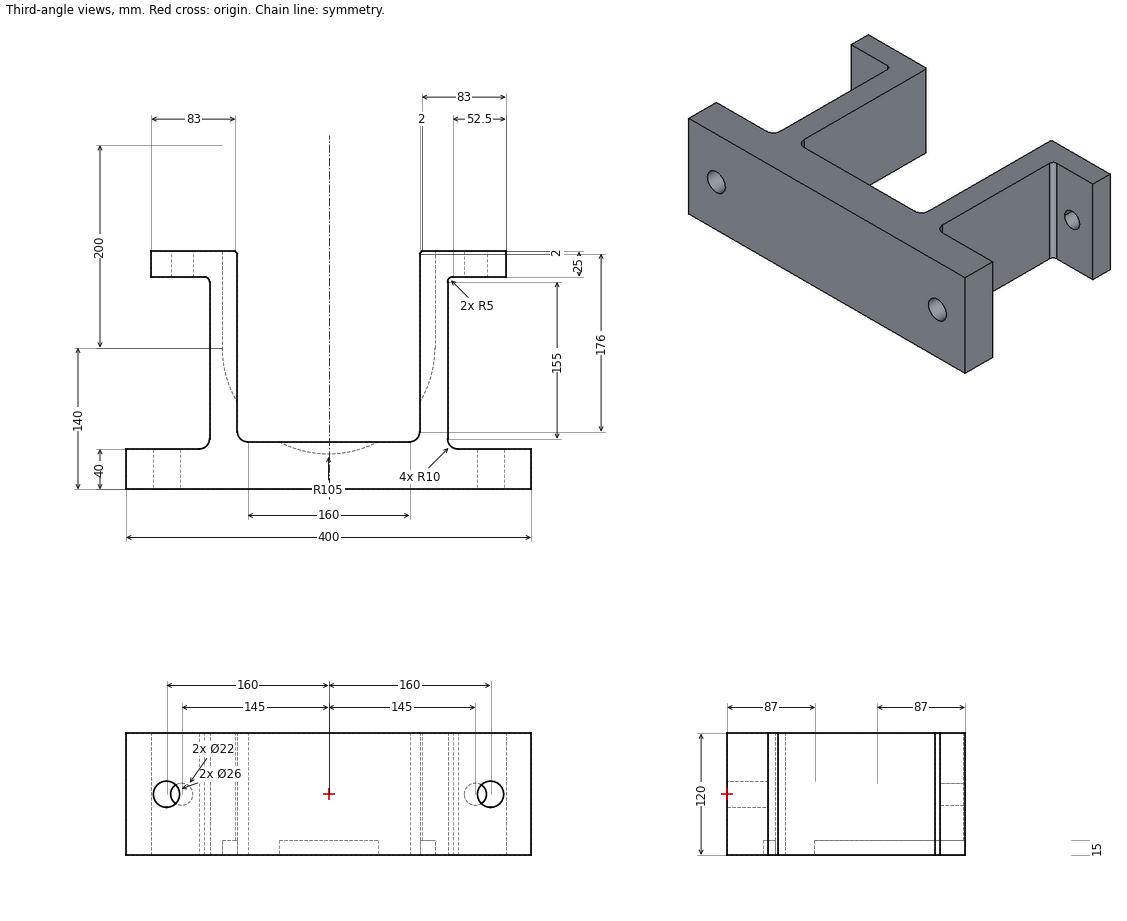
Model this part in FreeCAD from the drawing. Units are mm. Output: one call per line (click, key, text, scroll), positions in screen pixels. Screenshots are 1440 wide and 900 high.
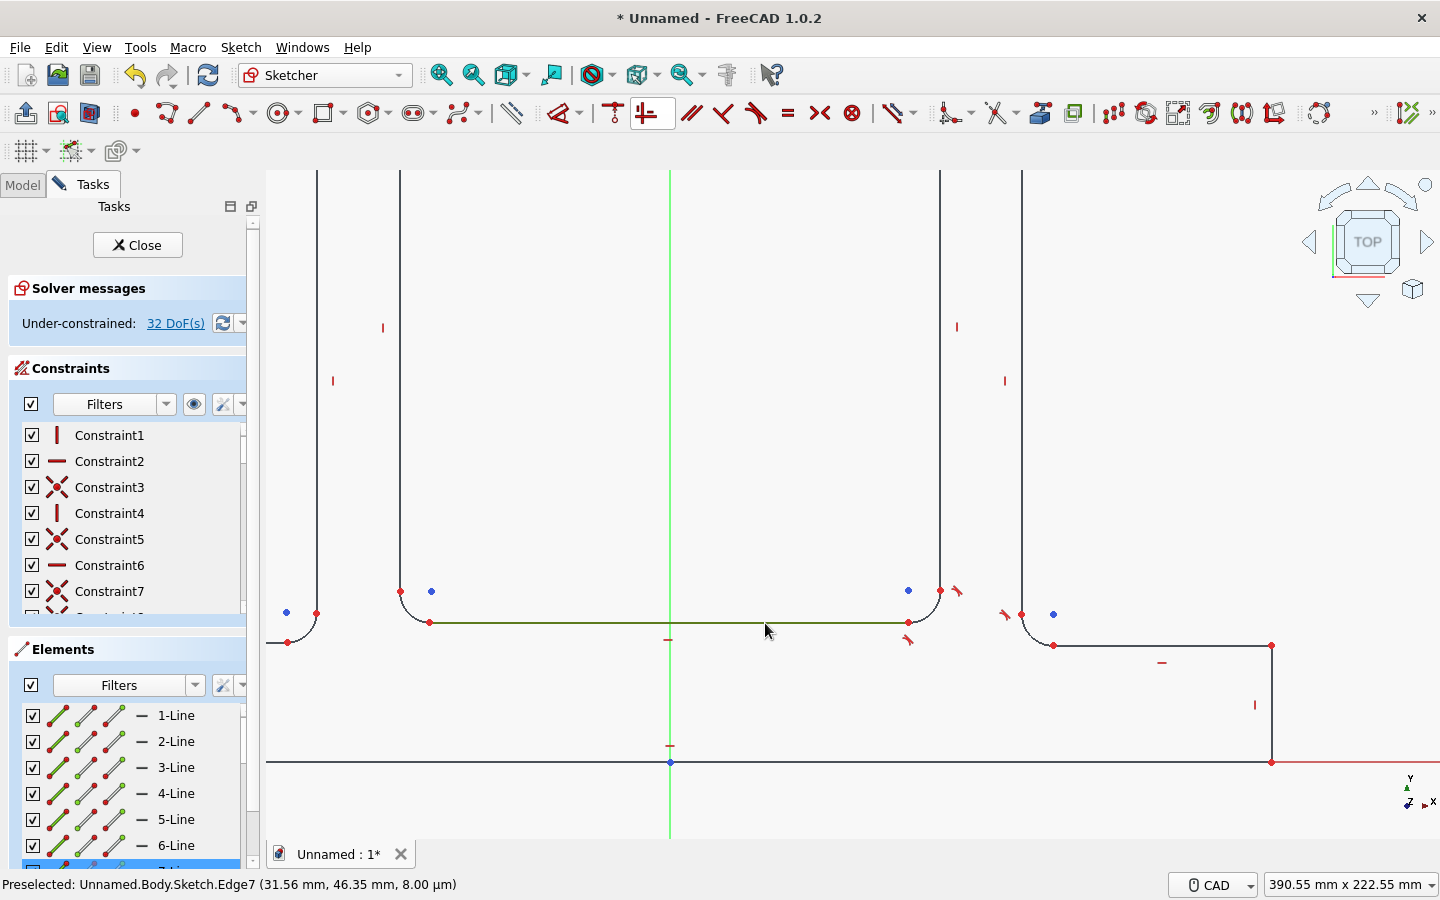
click(403, 605)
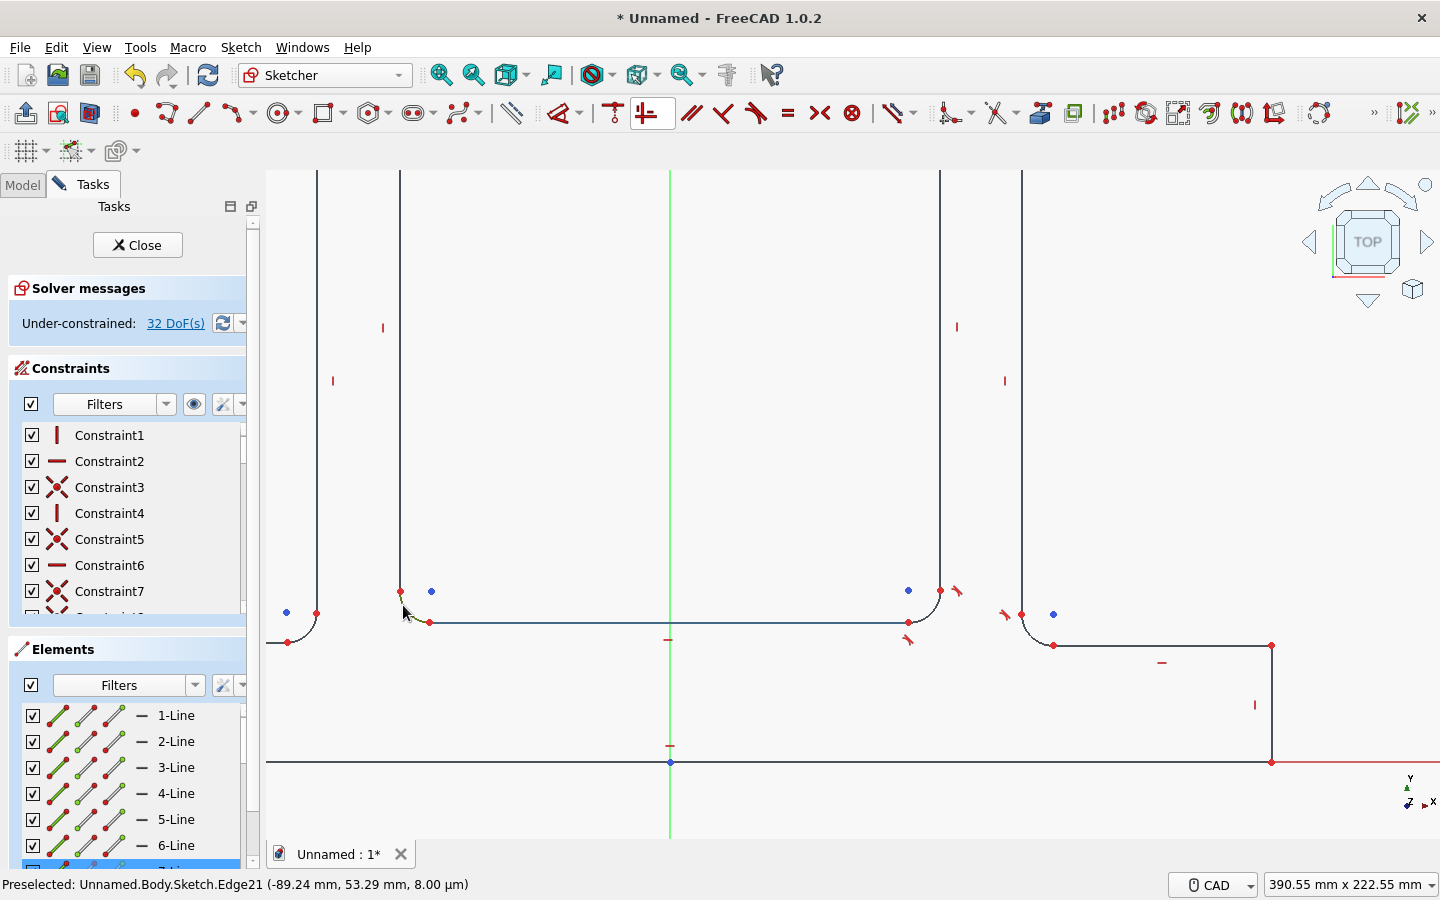
click(756, 114)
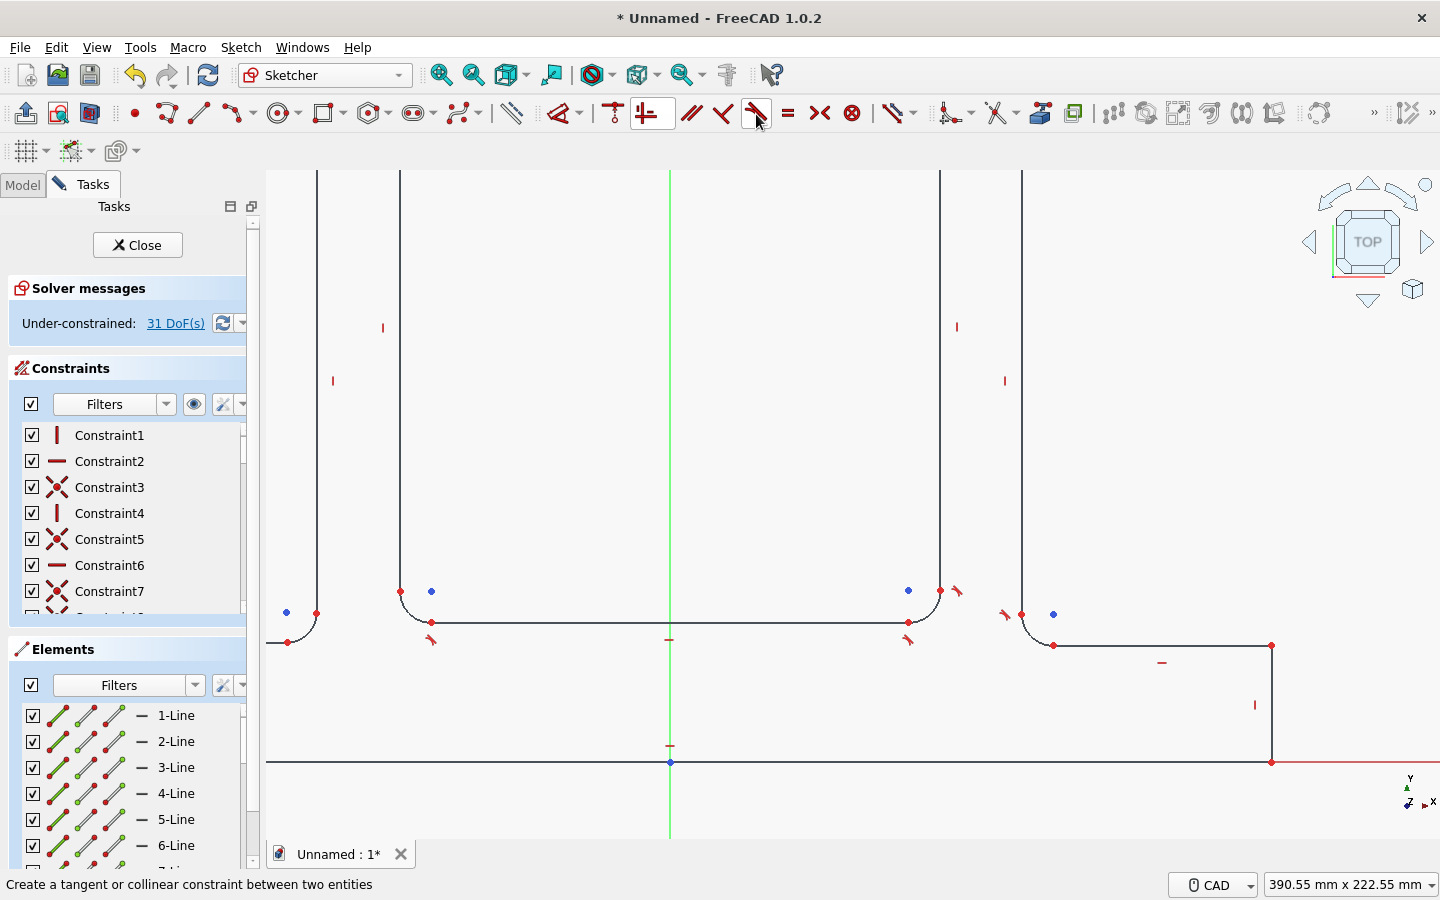
click(400, 433)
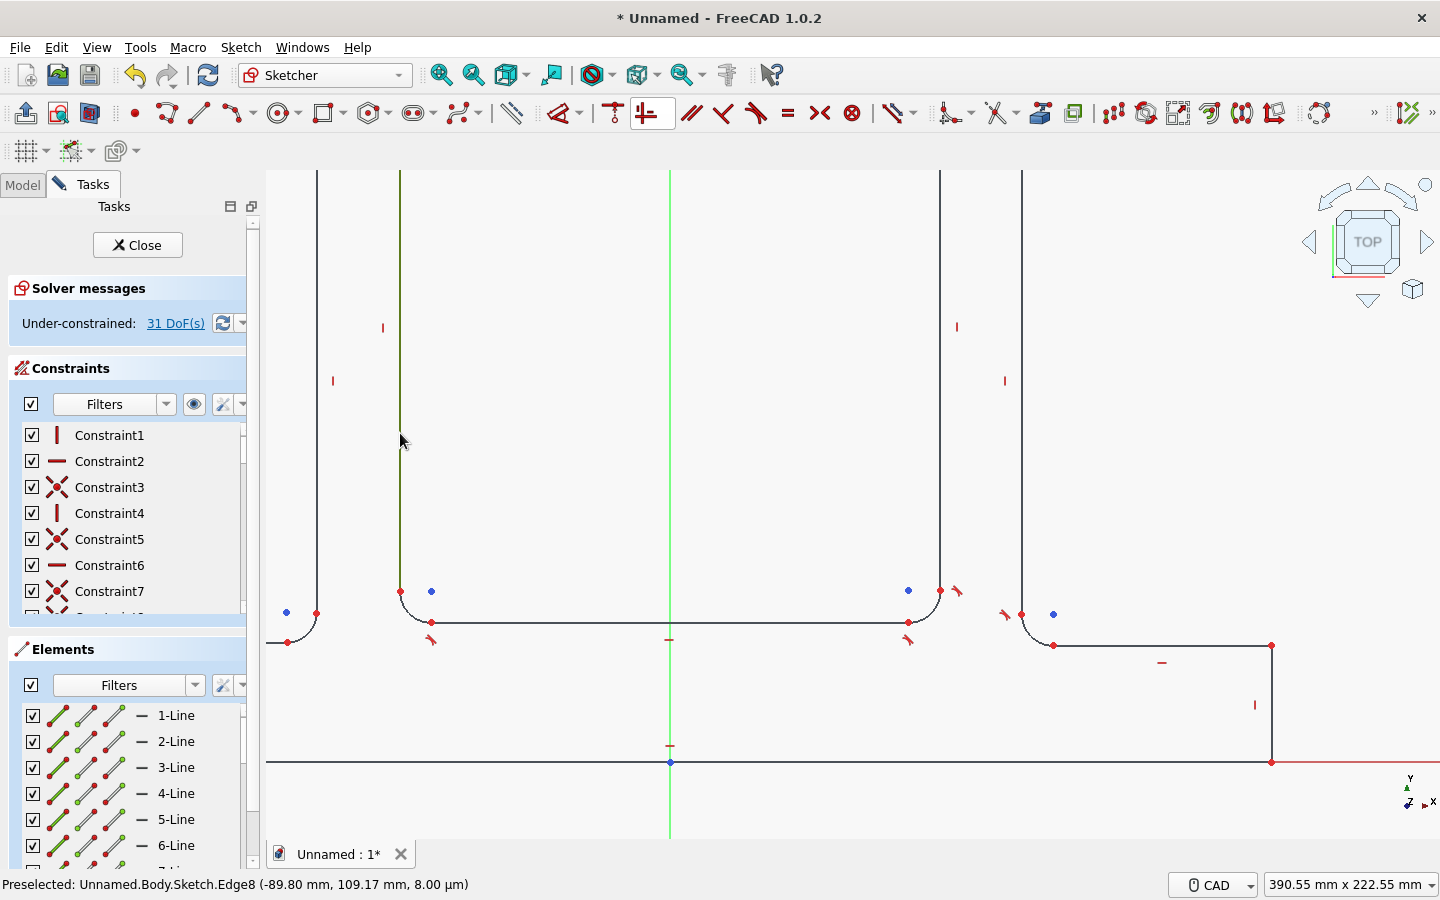
click(404, 606)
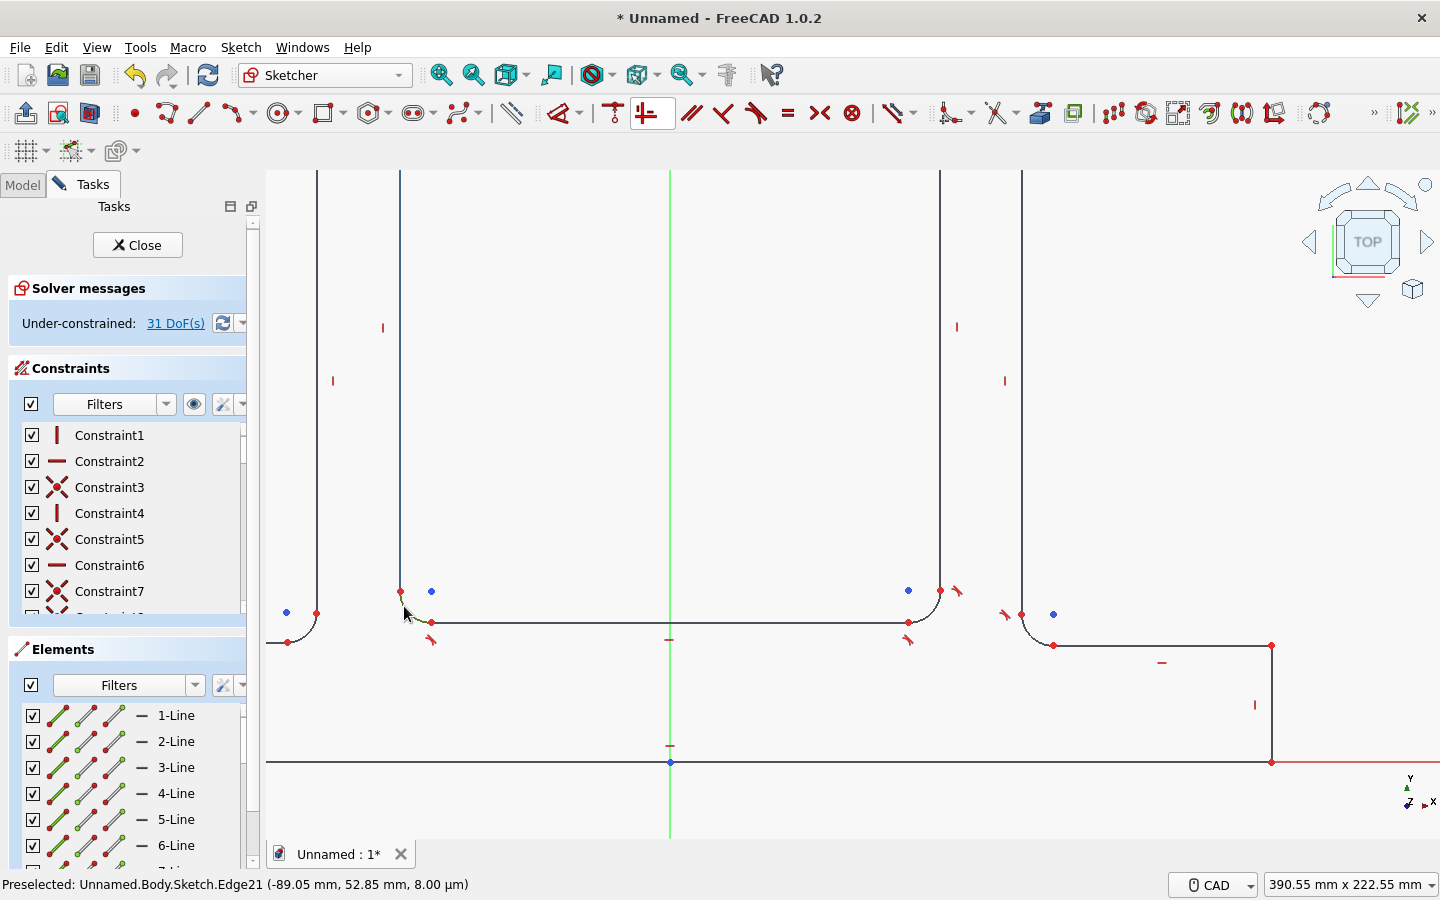
click(756, 114)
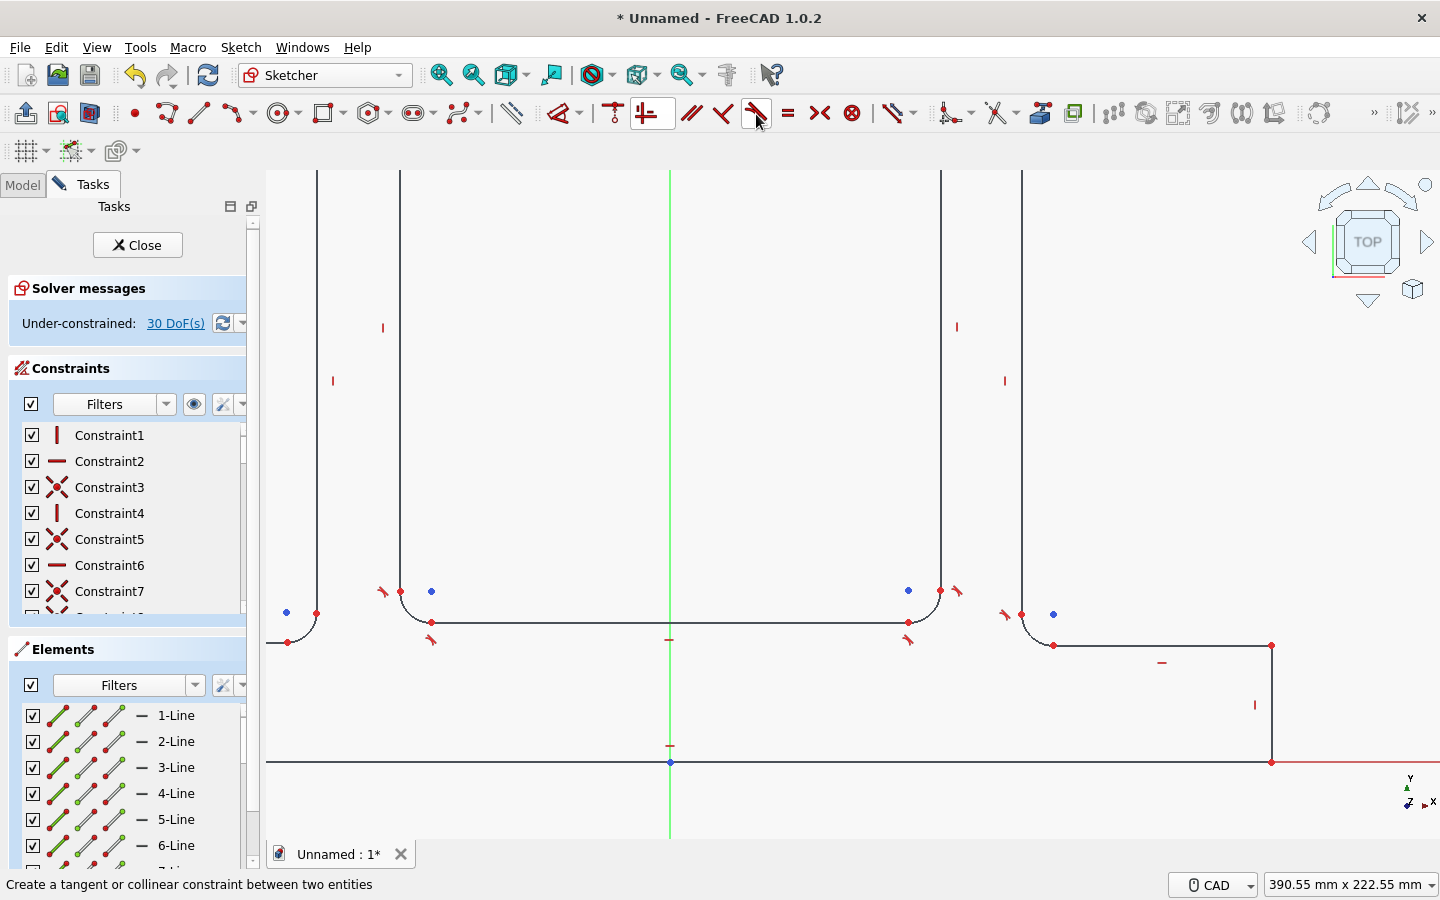
scroll(924, 621, down, 3)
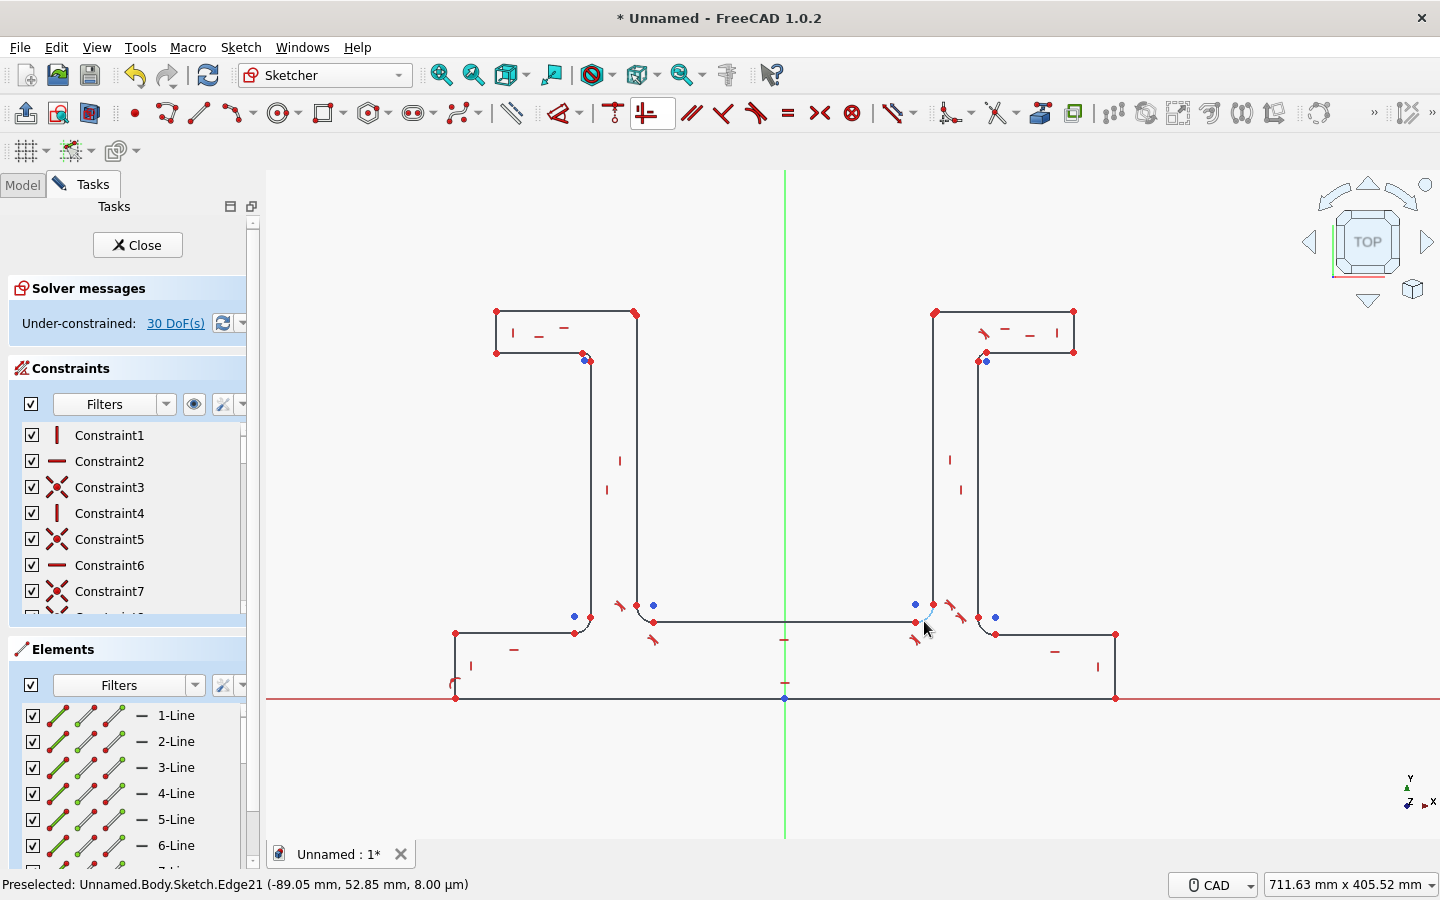
click(522, 353)